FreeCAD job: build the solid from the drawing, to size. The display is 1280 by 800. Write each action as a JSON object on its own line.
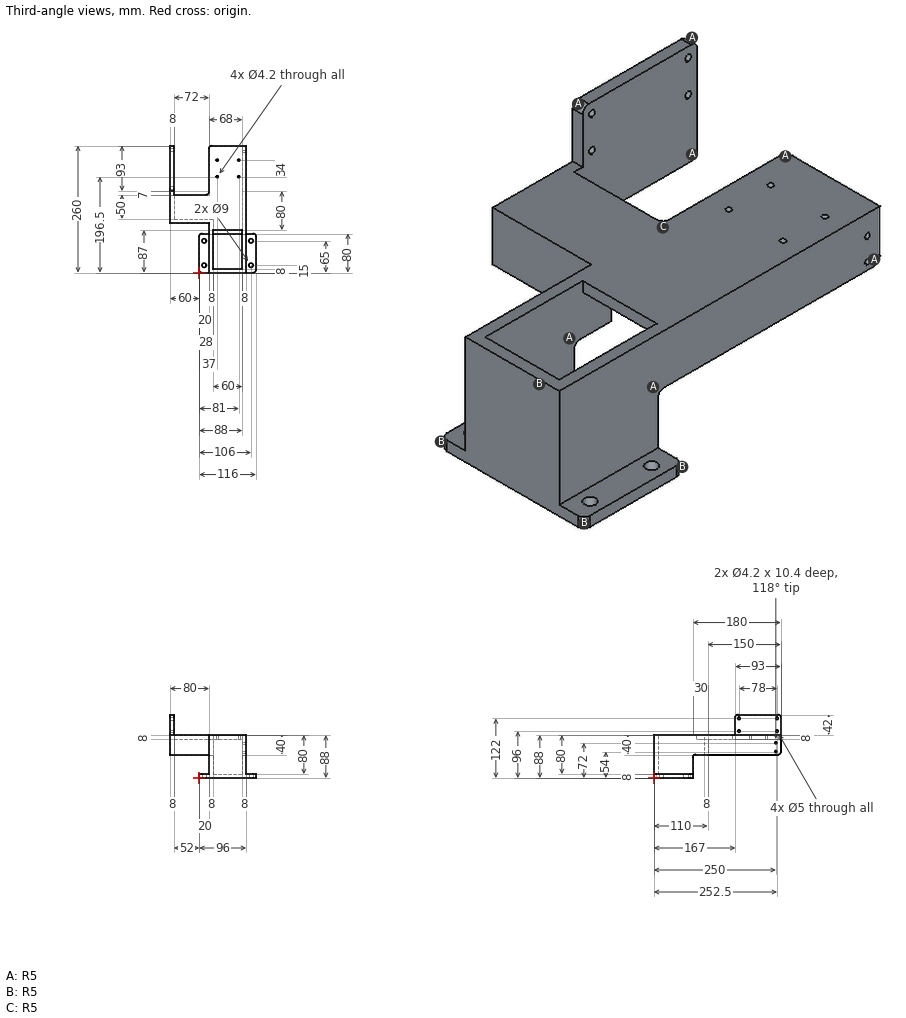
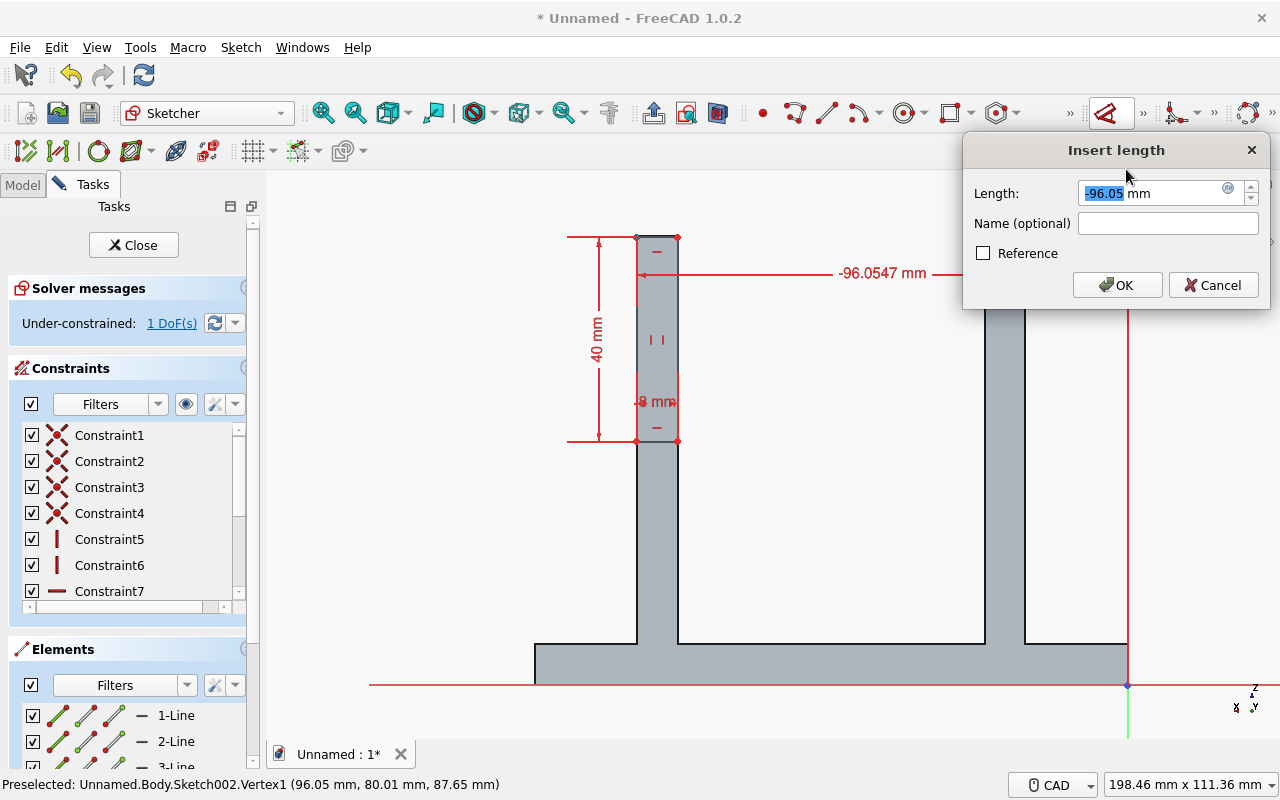
{"action": "type", "text": "-96"}
{"action": "key", "text": "Return"}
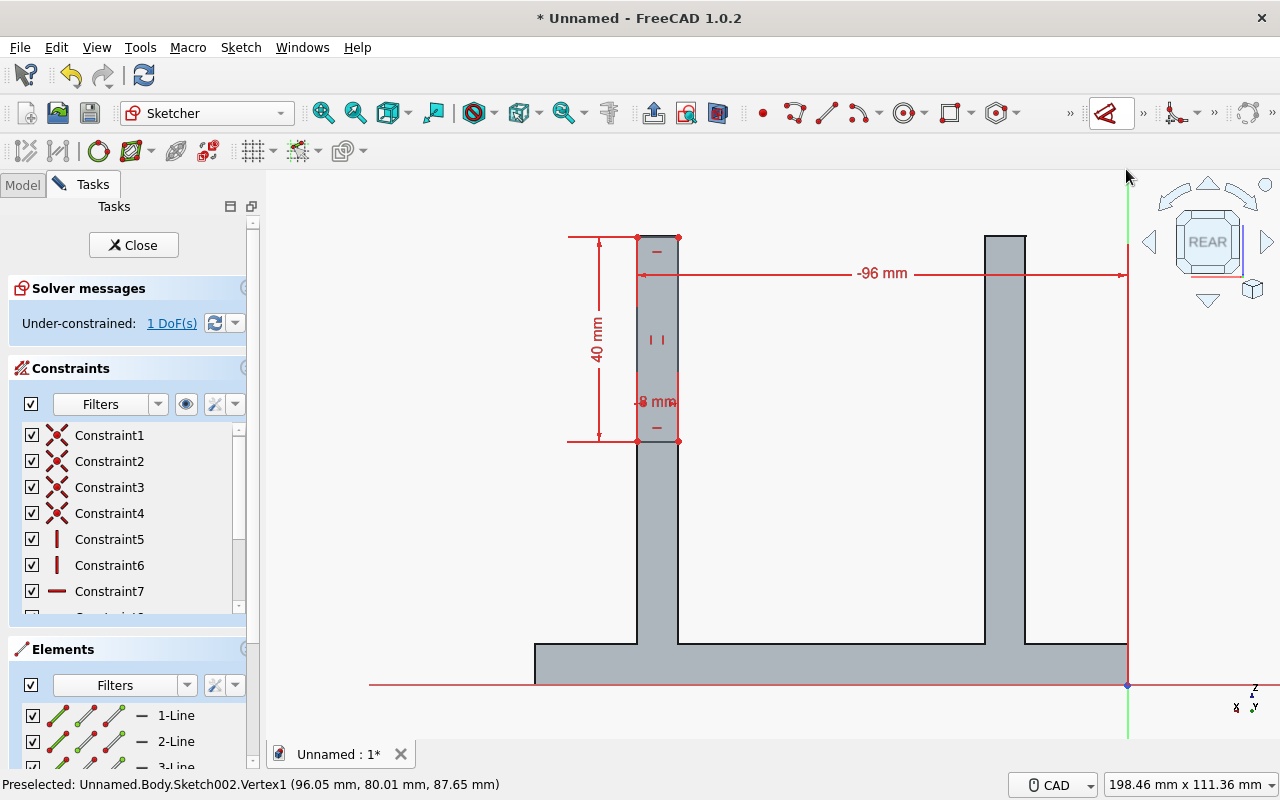
{"action": "left_click", "coordinate": [637, 237]}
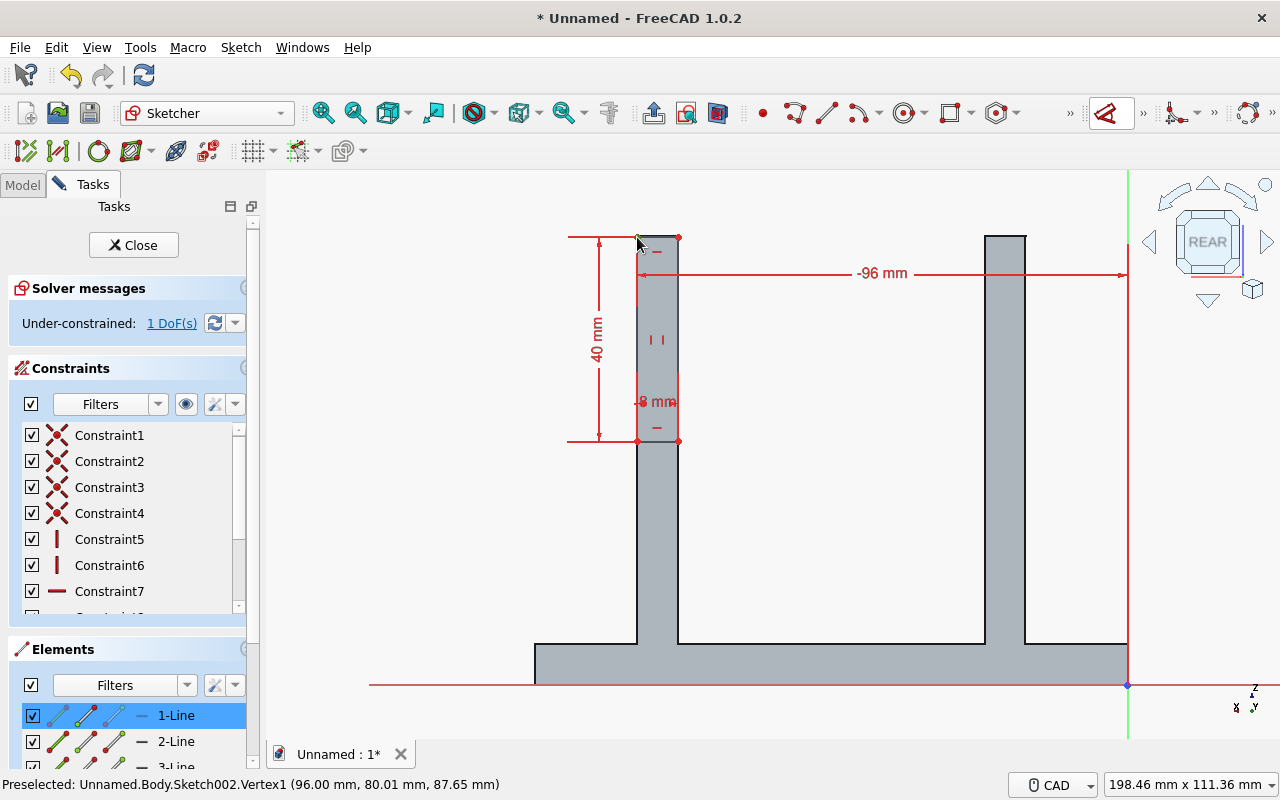
{"action": "left_click", "coordinate": [1128, 114]}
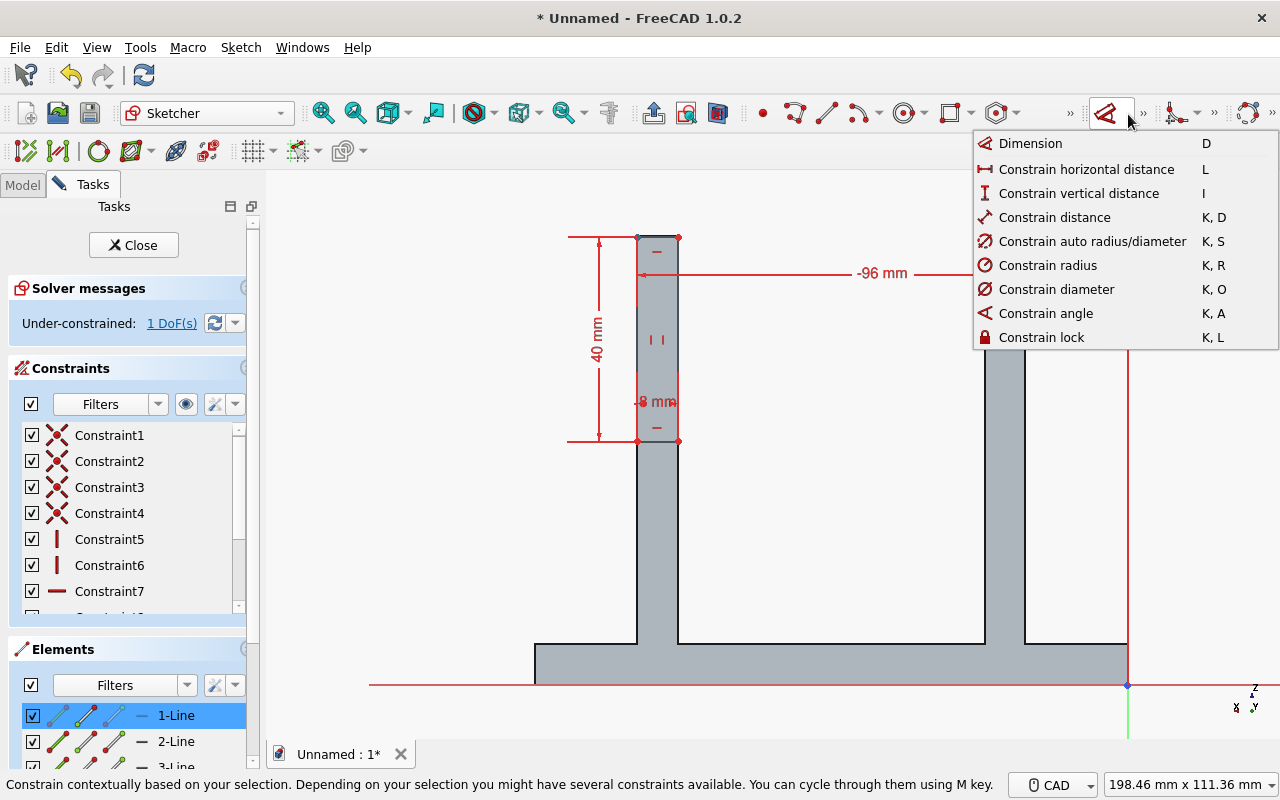
{"action": "left_click", "coordinate": [1126, 193]}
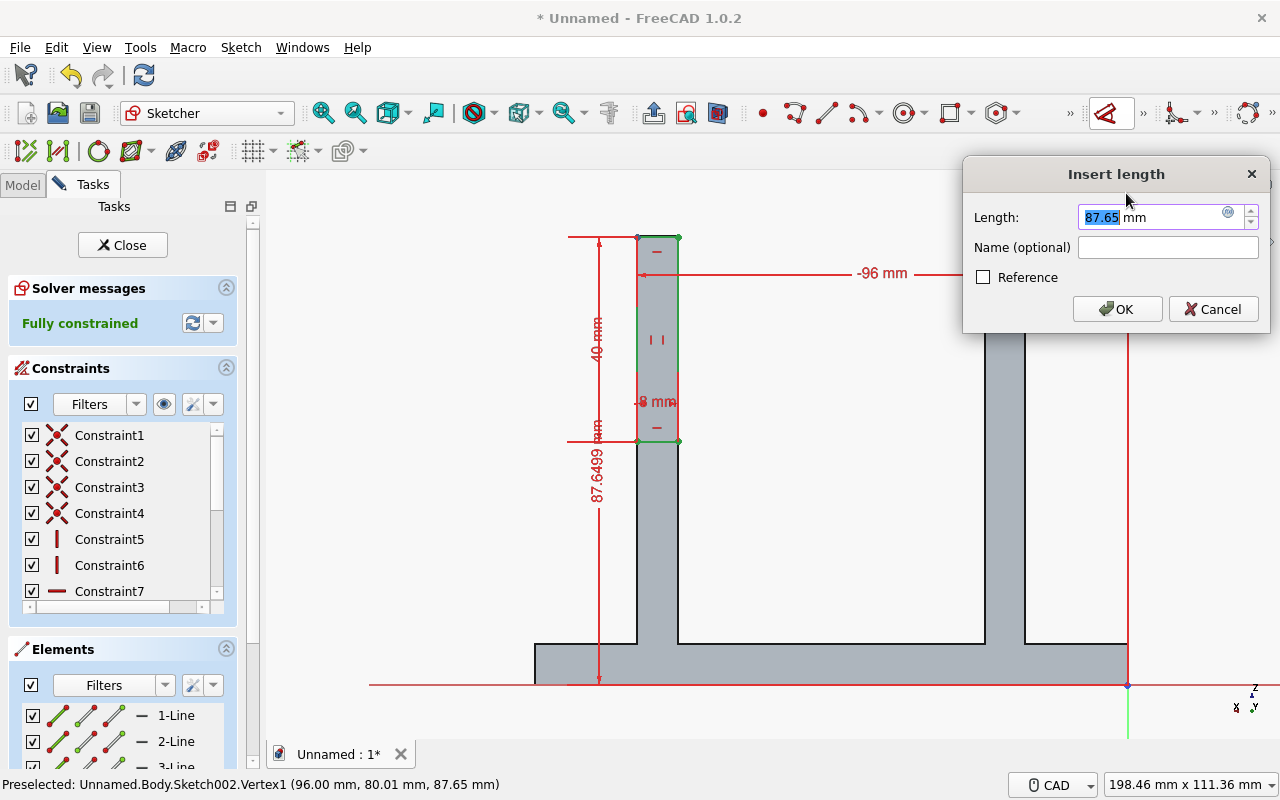
{"action": "type", "text": "88"}
{"action": "key", "text": "Return"}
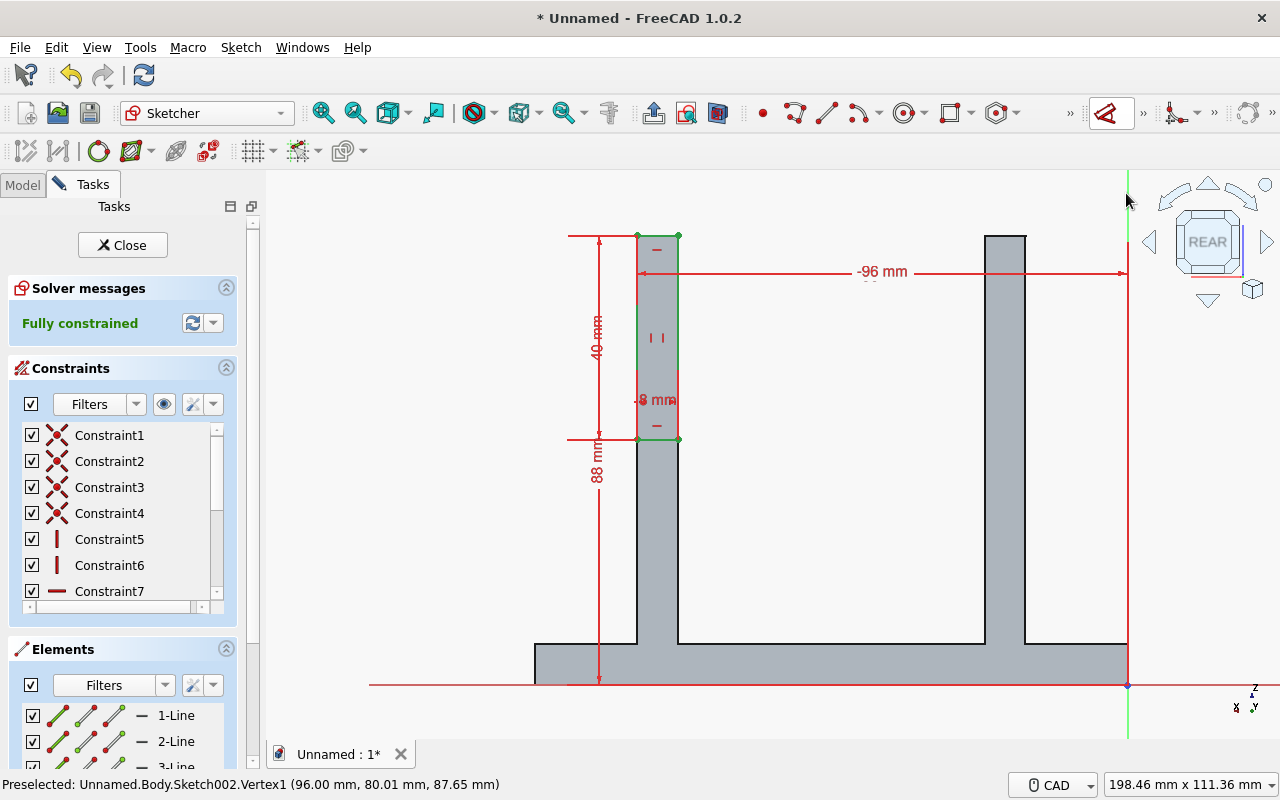
{"action": "left_click", "coordinate": [123, 245]}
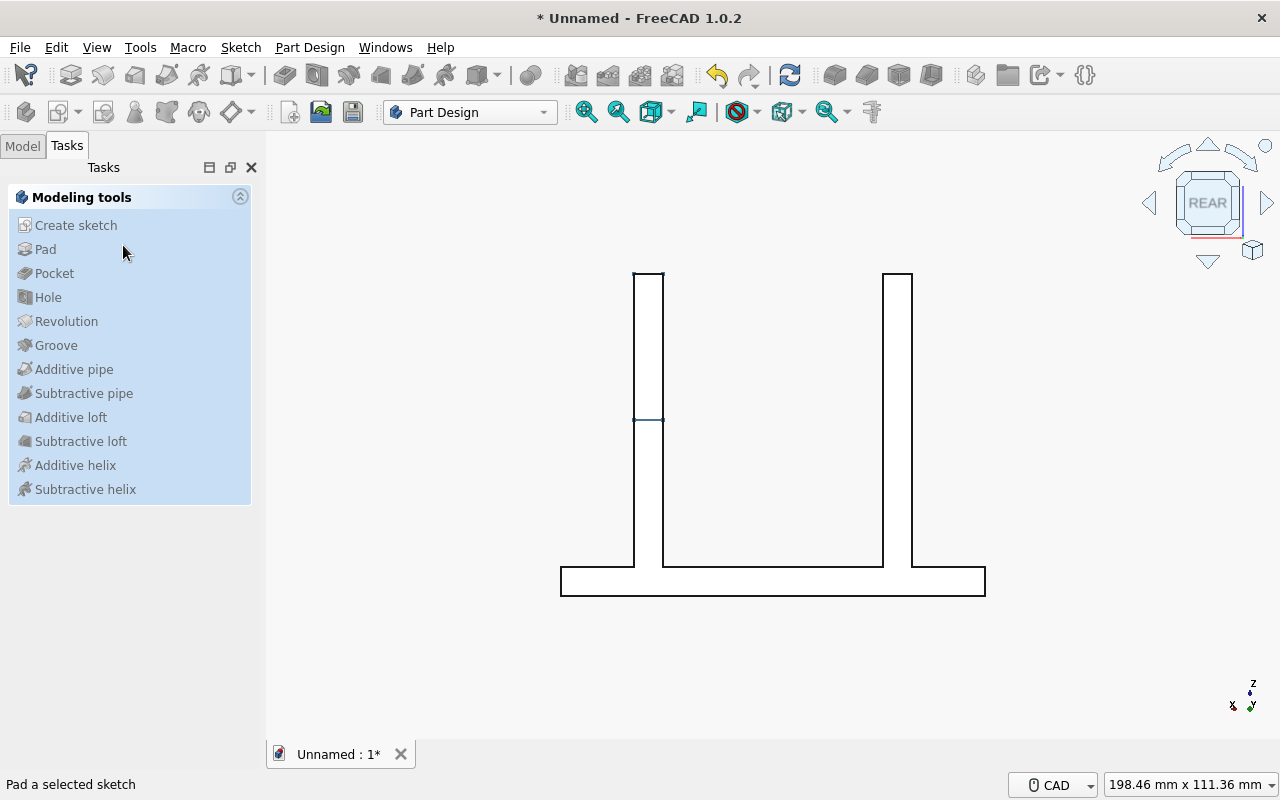
{"action": "left_click", "coordinate": [72, 76]}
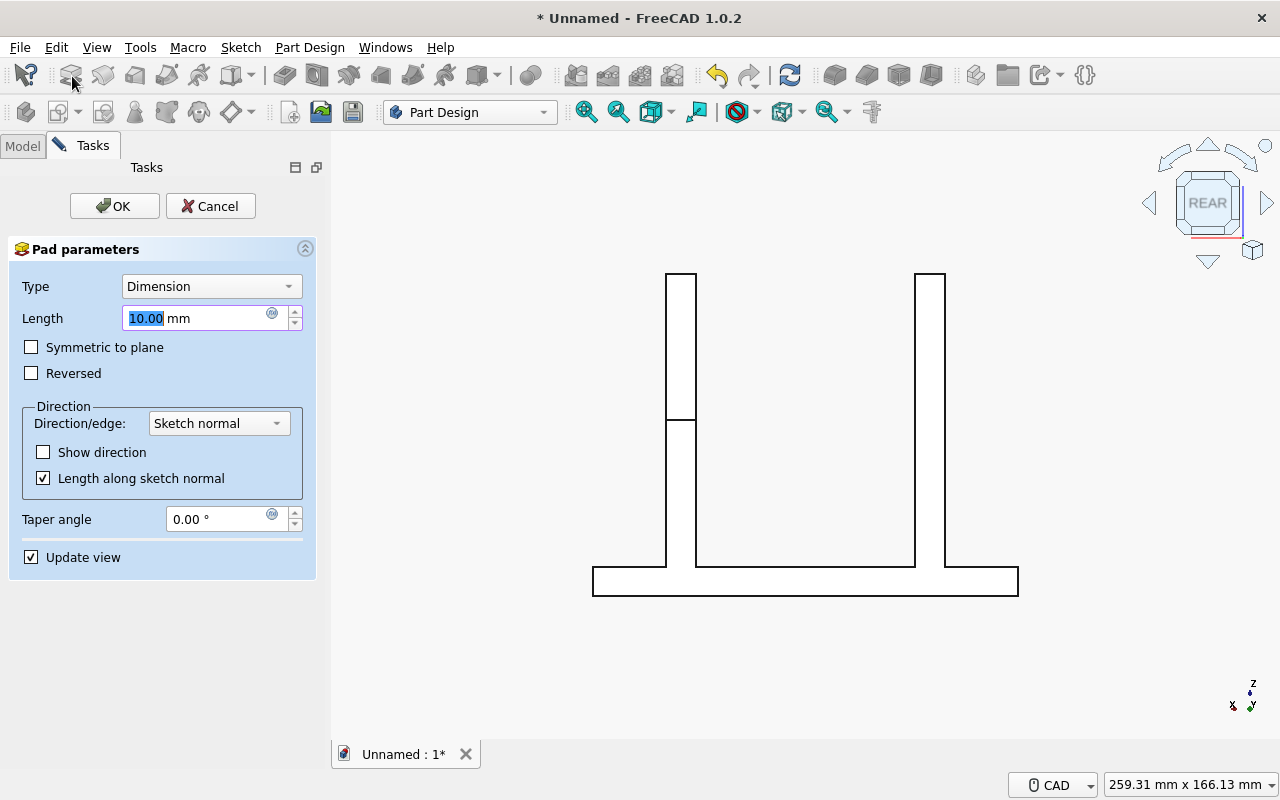
{"action": "type", "text": "180"}
{"action": "key", "text": "Tab"}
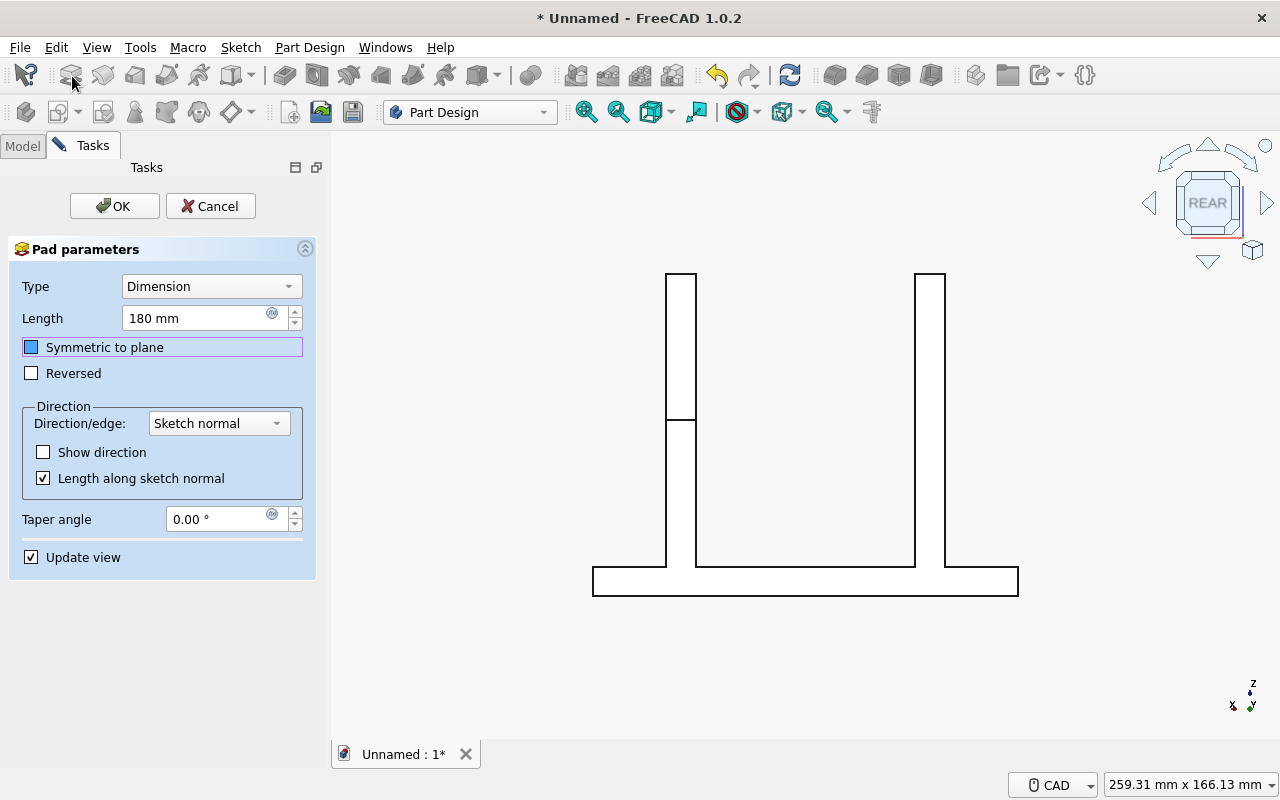
{"action": "left_click", "coordinate": [115, 206]}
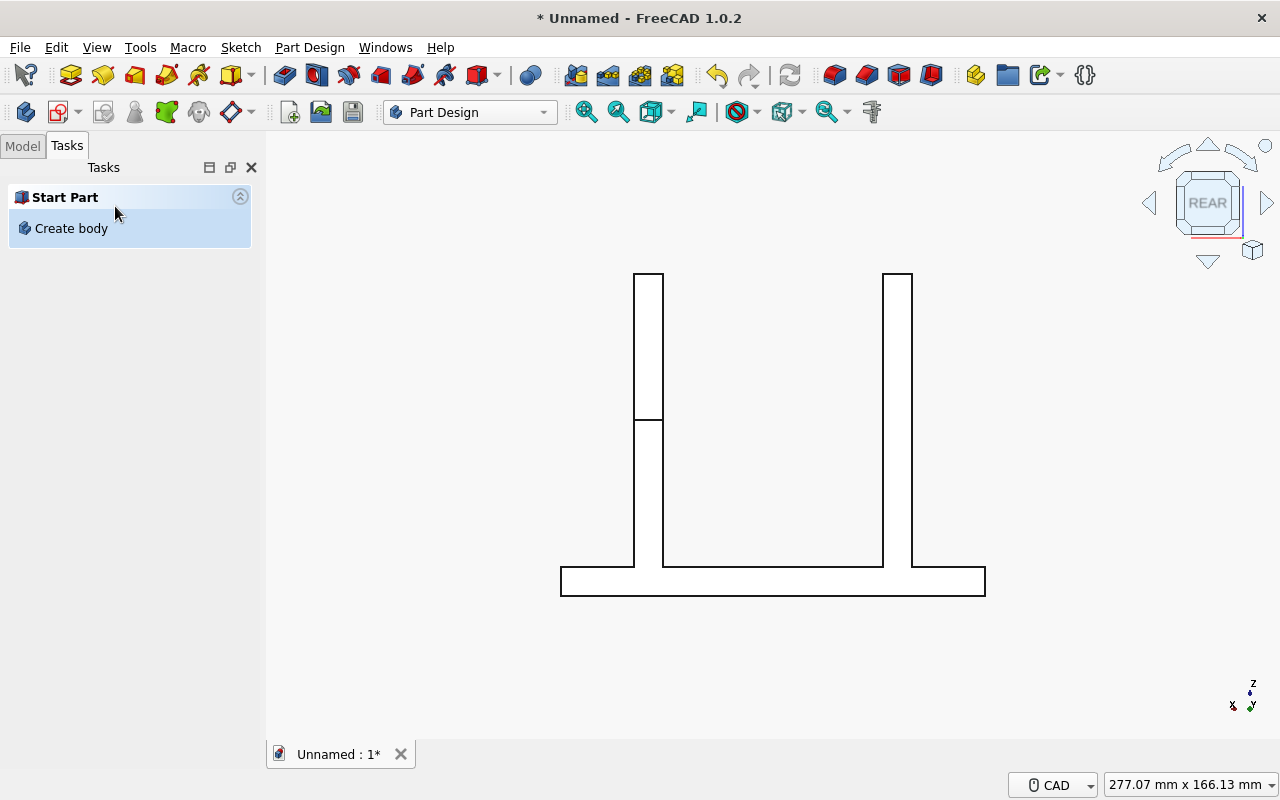
{"action": "key", "text": "0"}